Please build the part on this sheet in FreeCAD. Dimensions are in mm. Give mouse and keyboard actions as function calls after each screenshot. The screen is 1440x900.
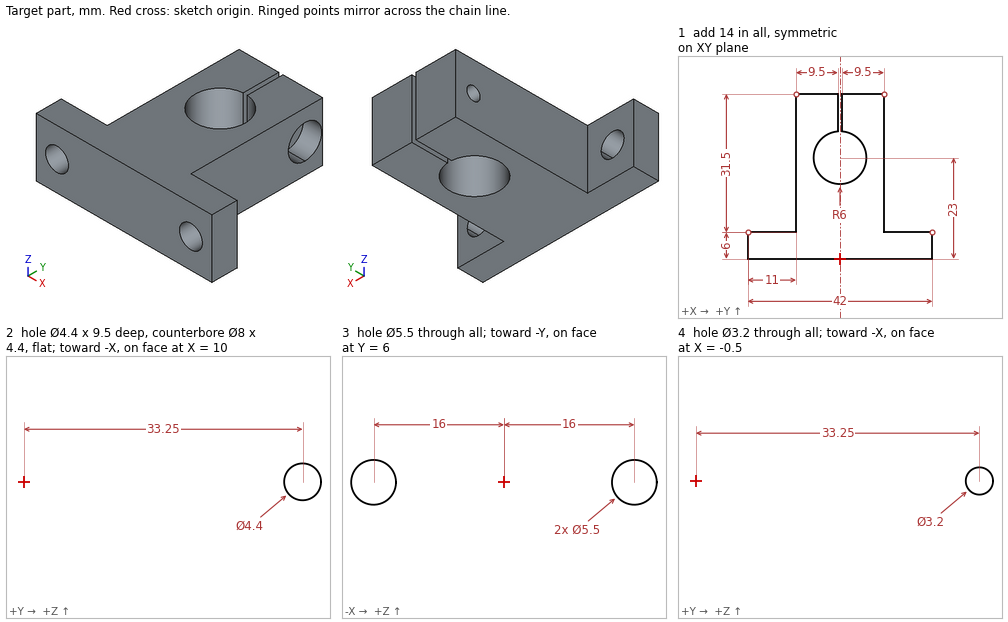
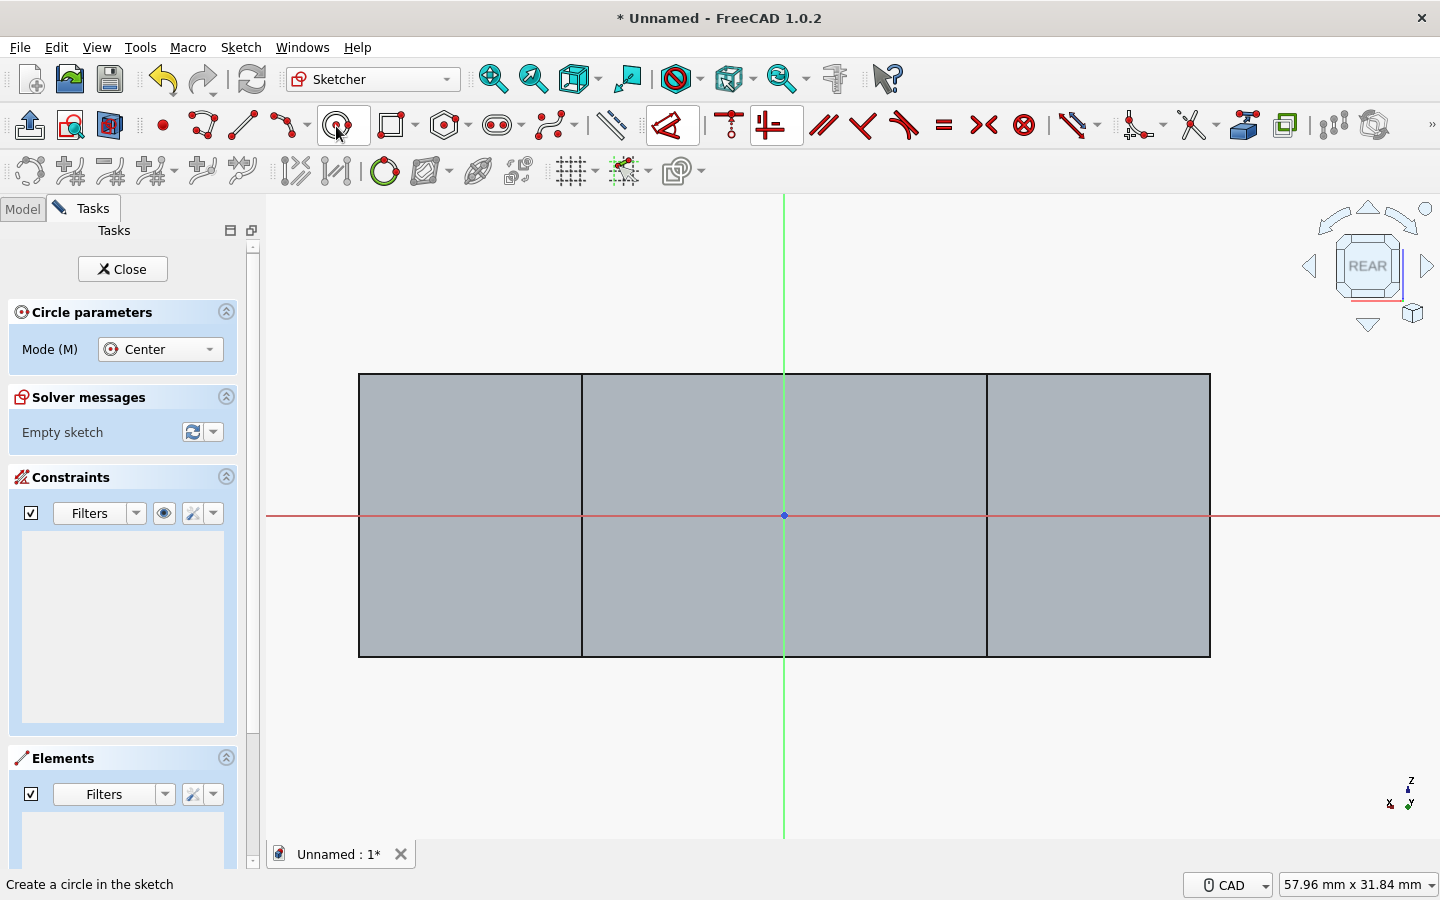
click(1108, 516)
click(1148, 476)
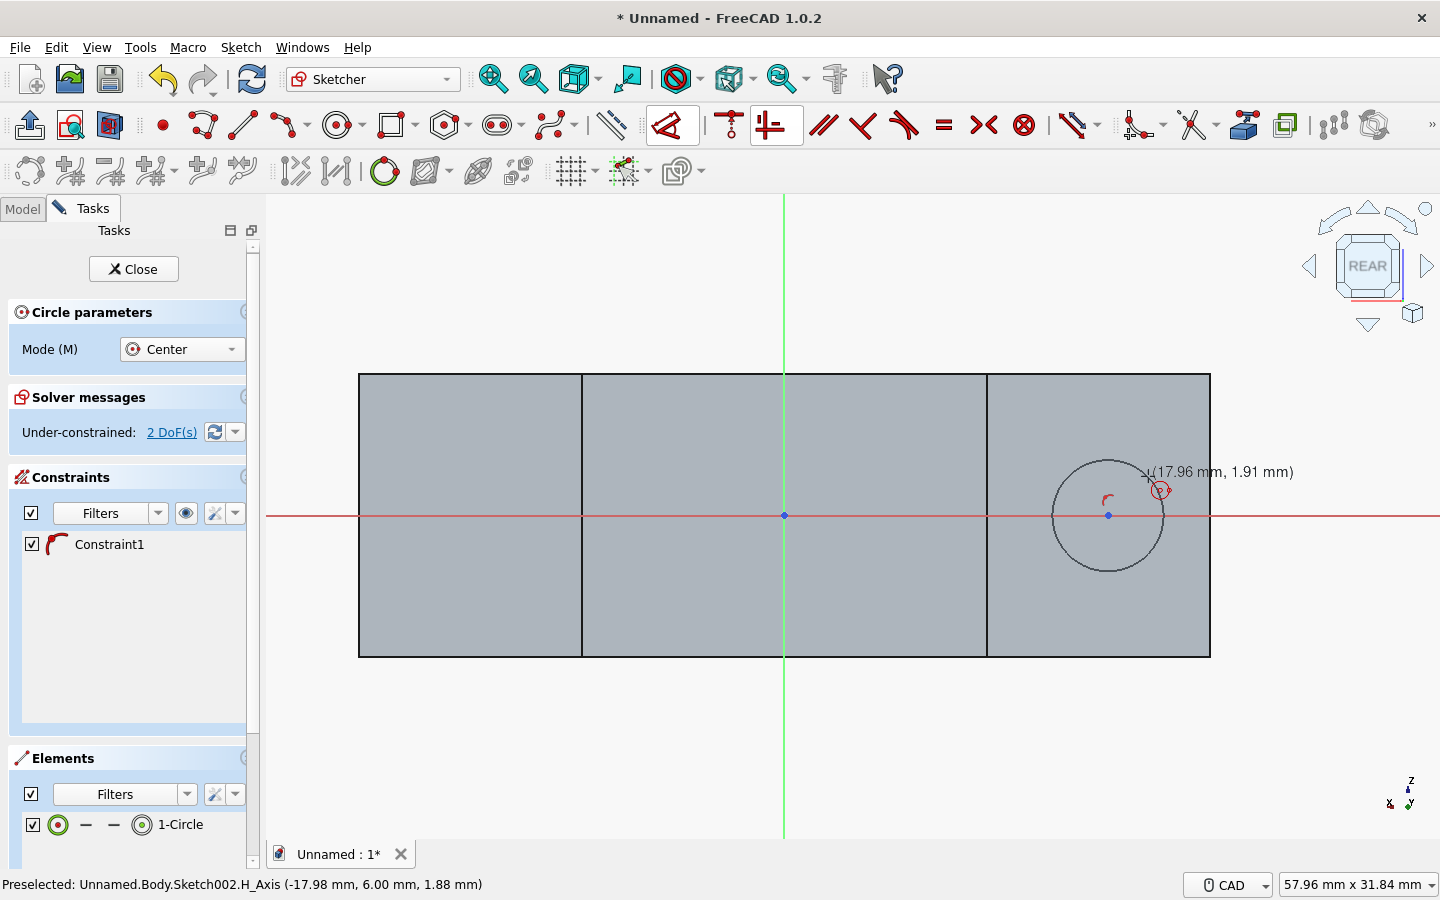
click(460, 516)
click(500, 476)
key(Escape)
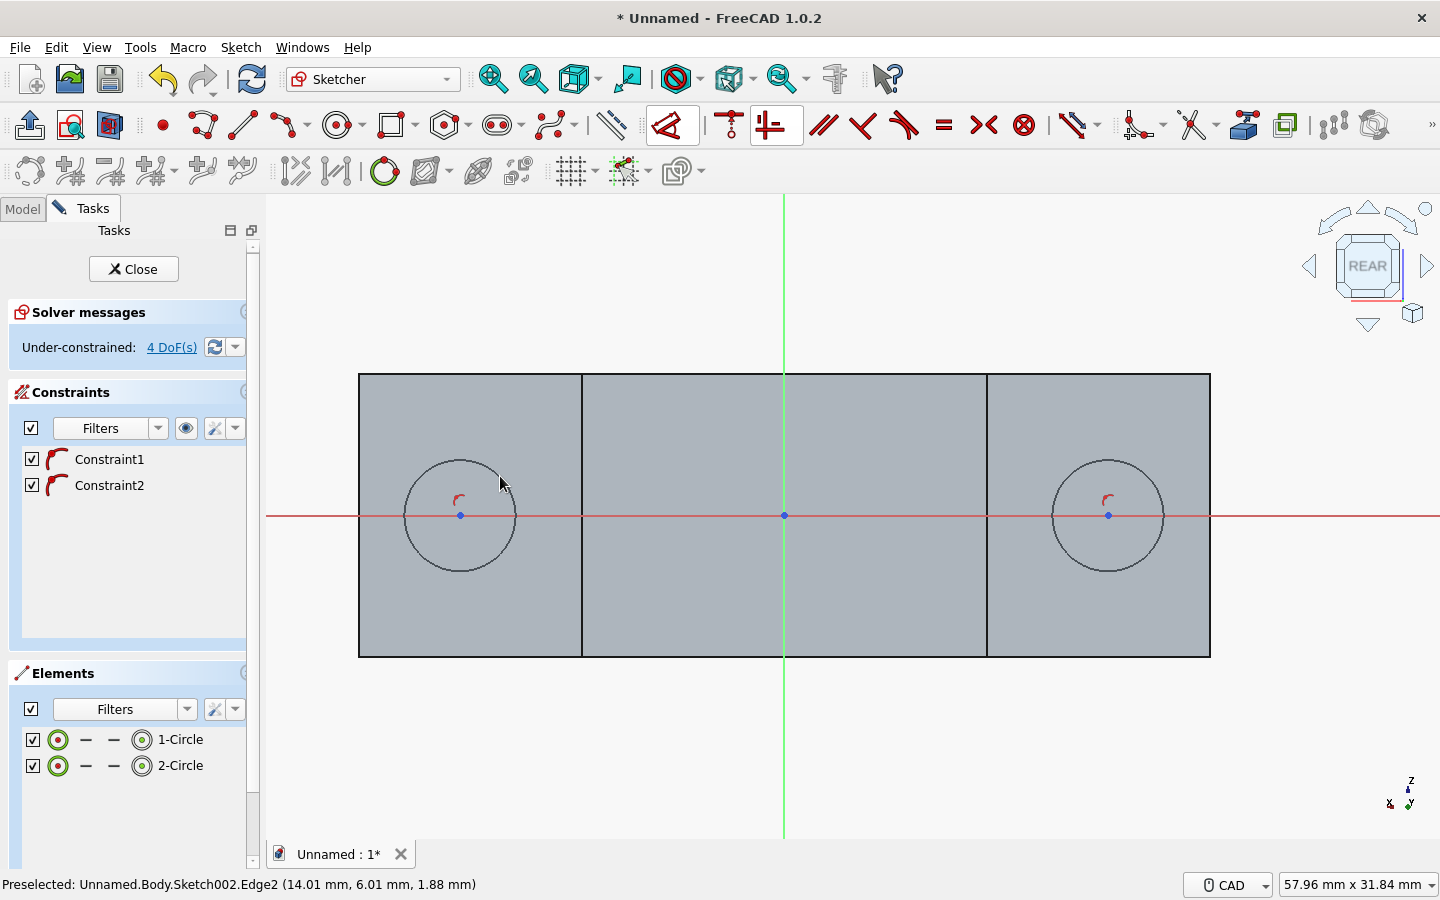
click(1147, 476)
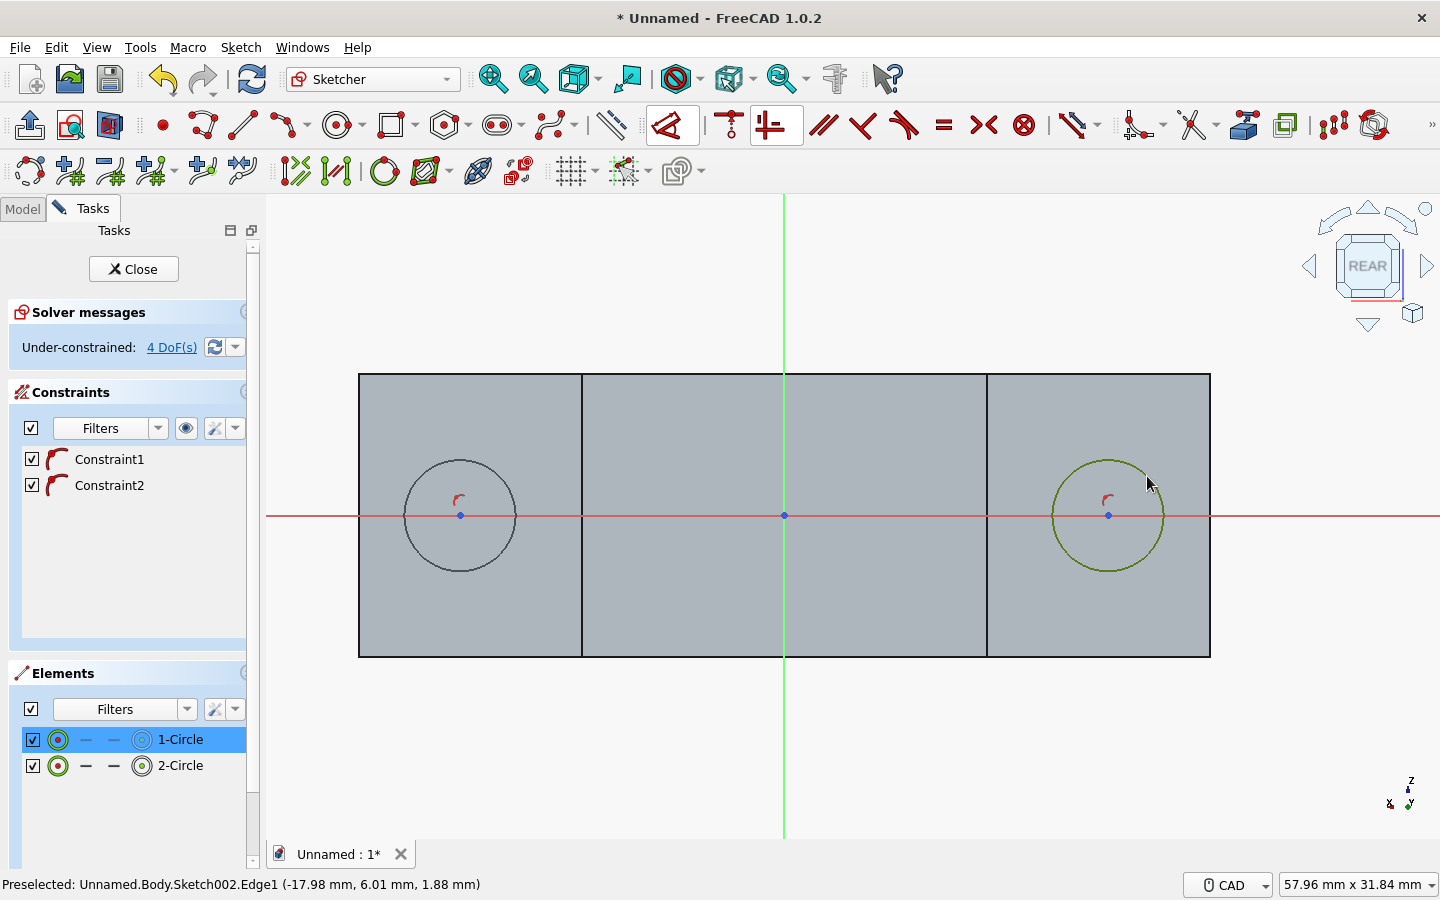
click(499, 476)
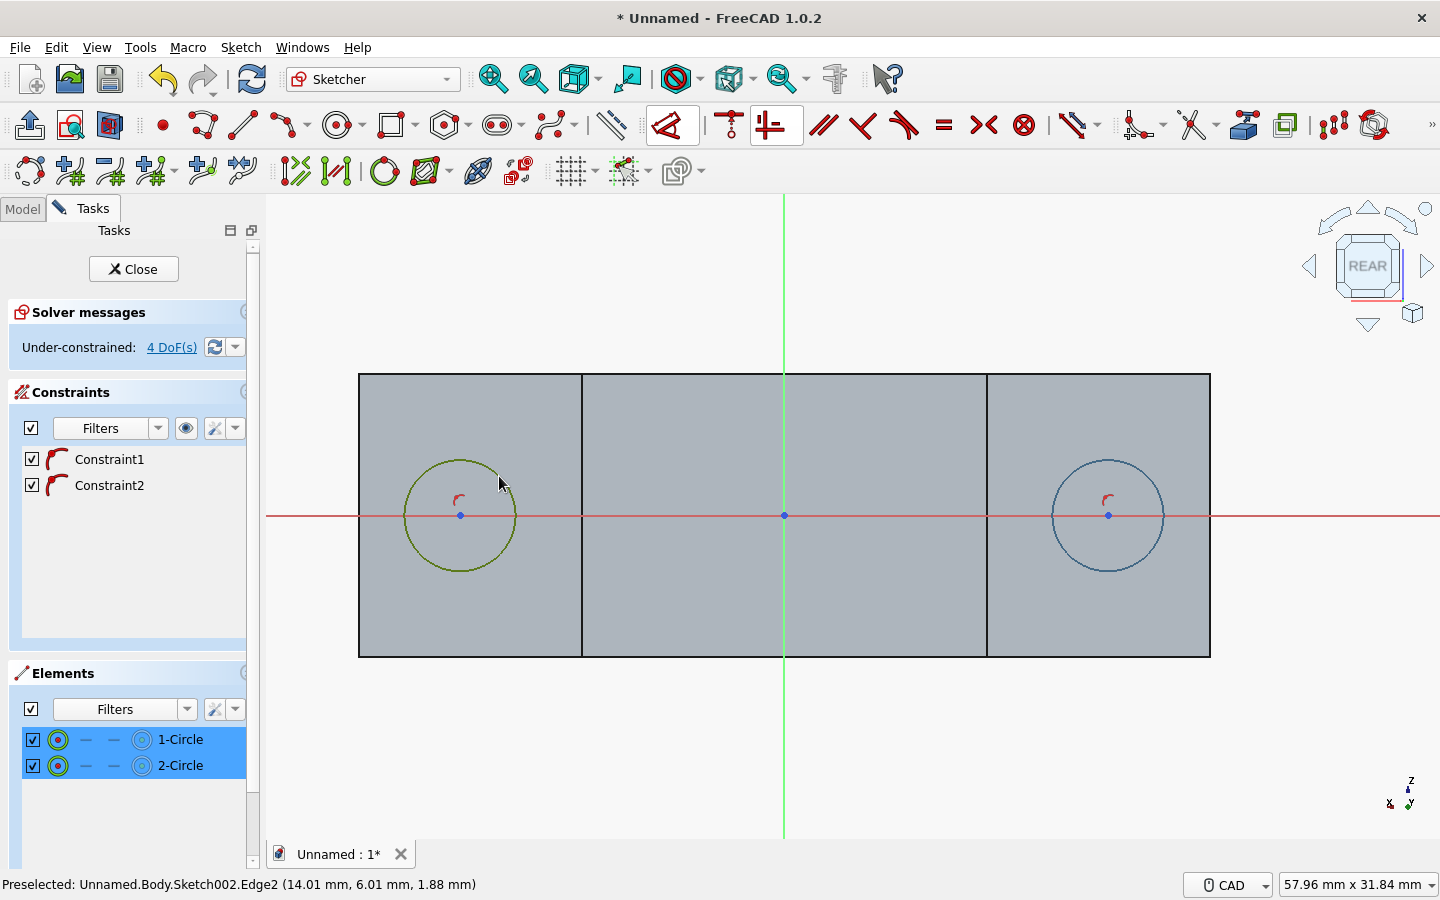
click(944, 126)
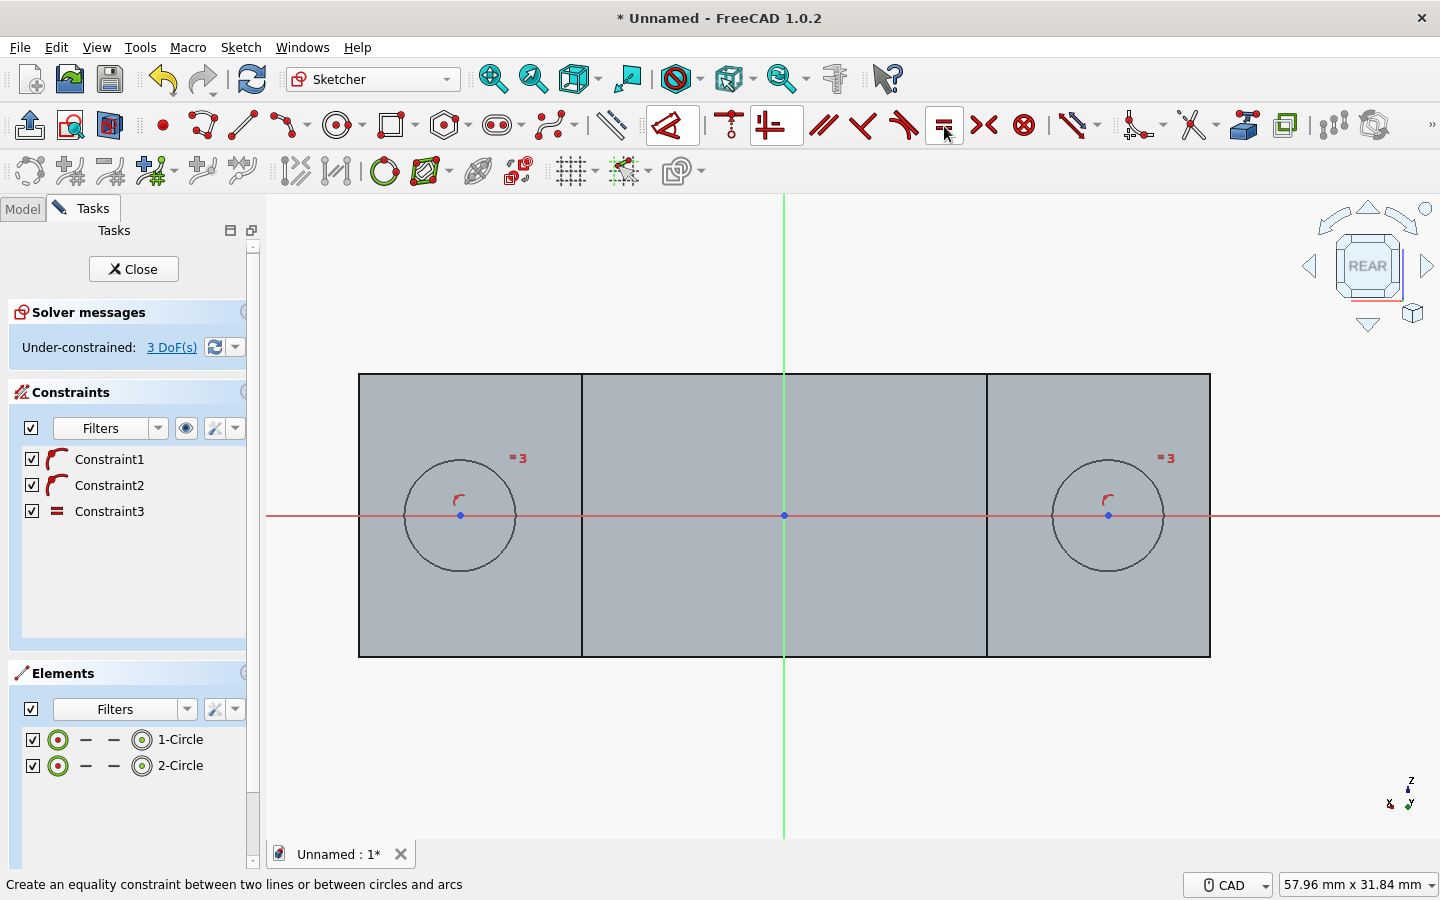
click(1147, 476)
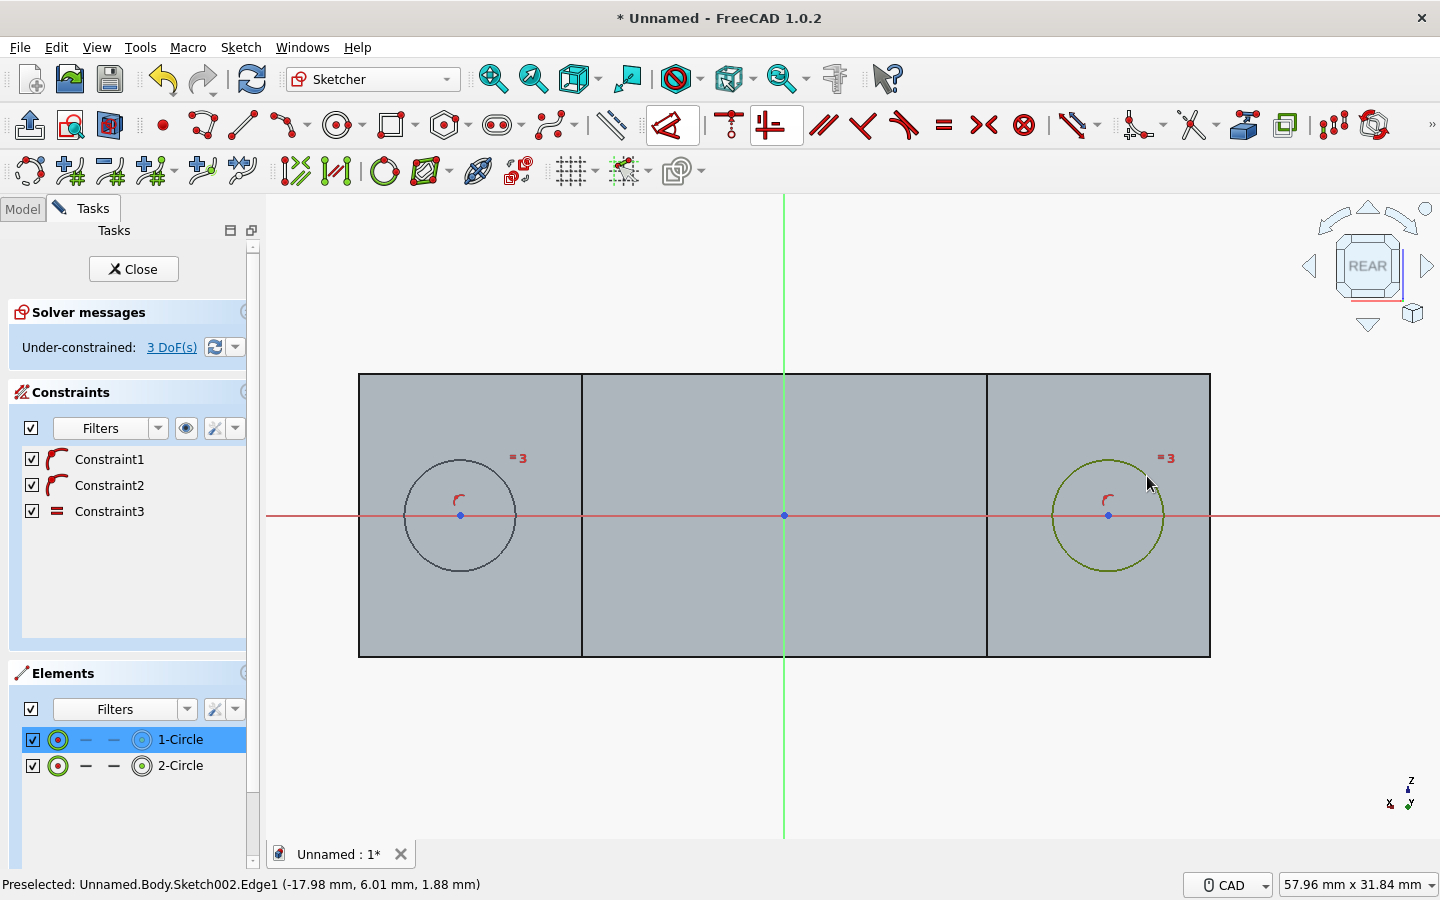
key(k)
key(o)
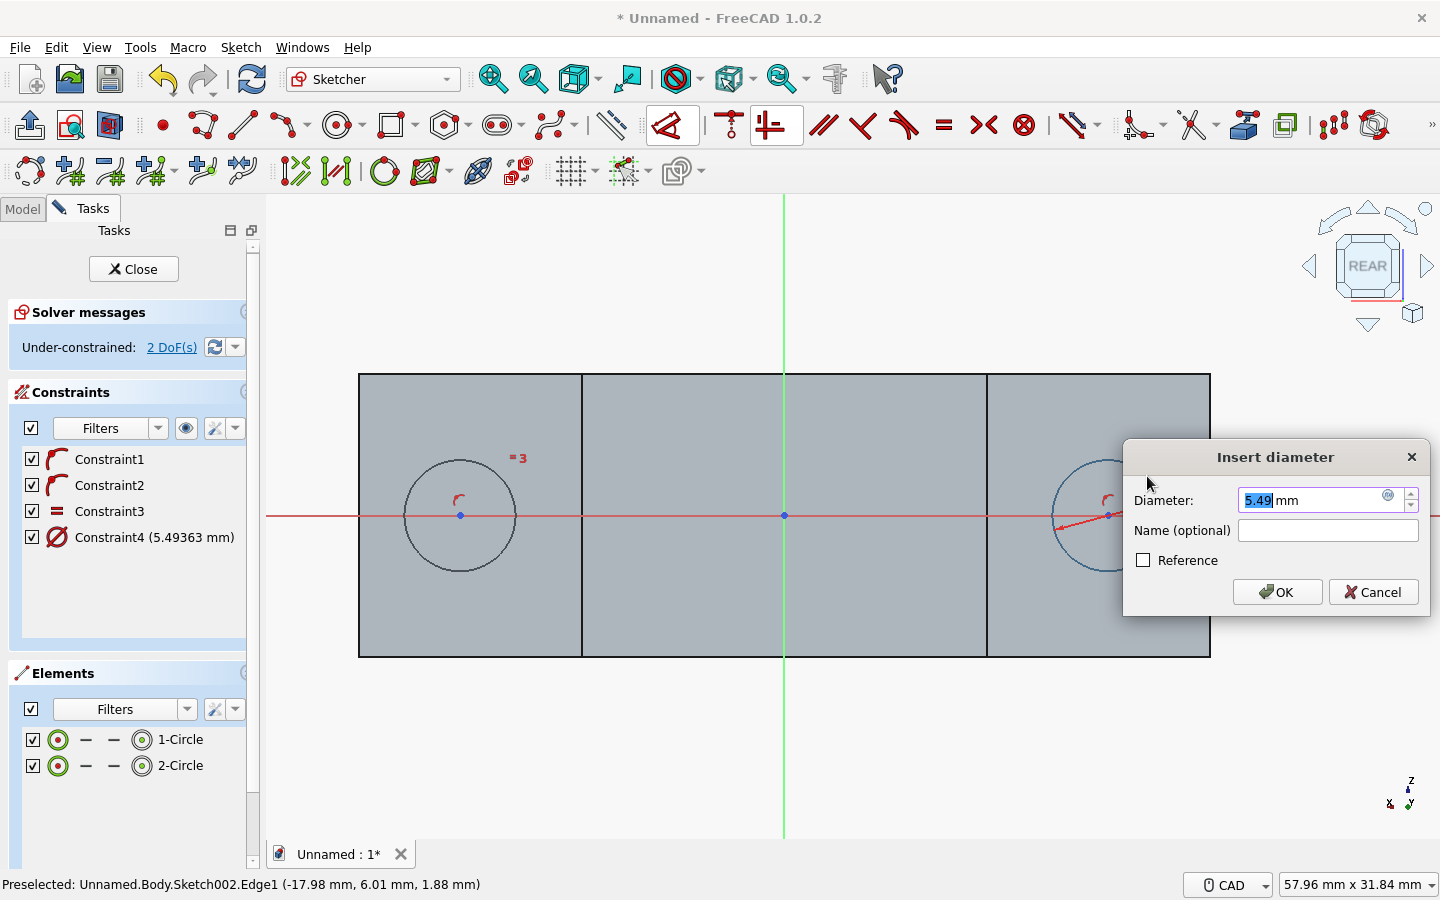
text(5.5)
key(Return)